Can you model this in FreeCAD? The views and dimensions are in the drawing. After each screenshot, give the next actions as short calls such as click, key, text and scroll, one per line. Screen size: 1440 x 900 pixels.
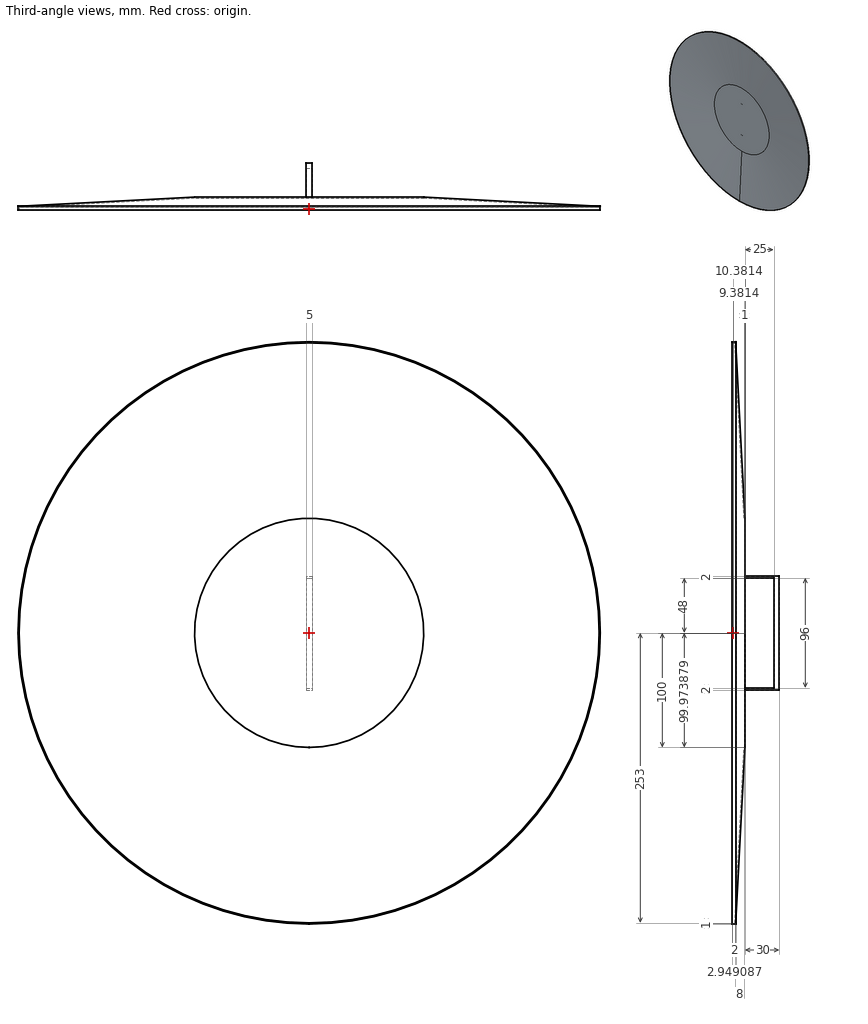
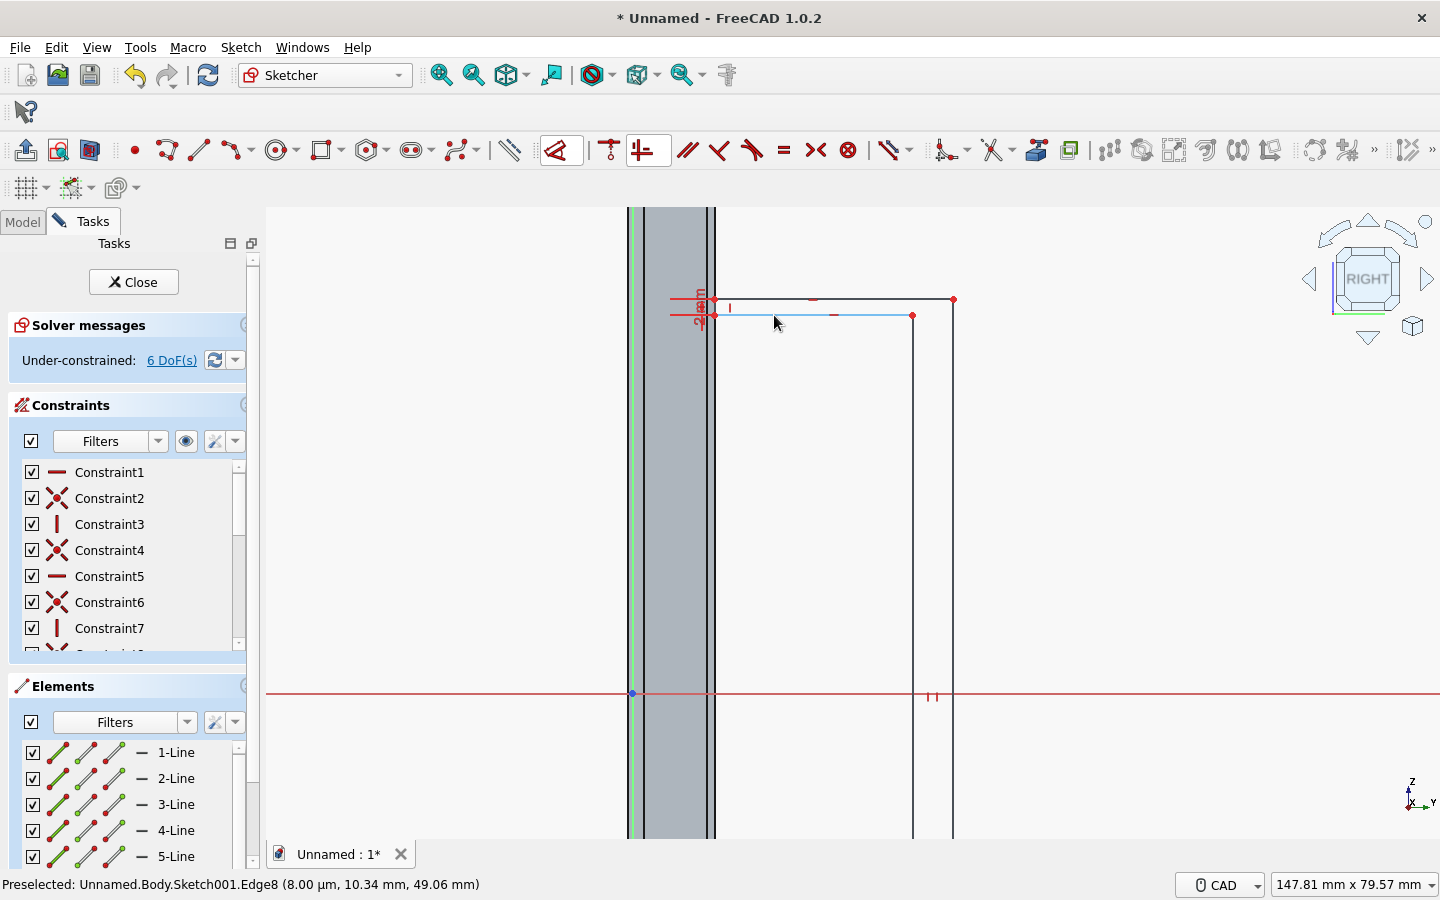
click(774, 315)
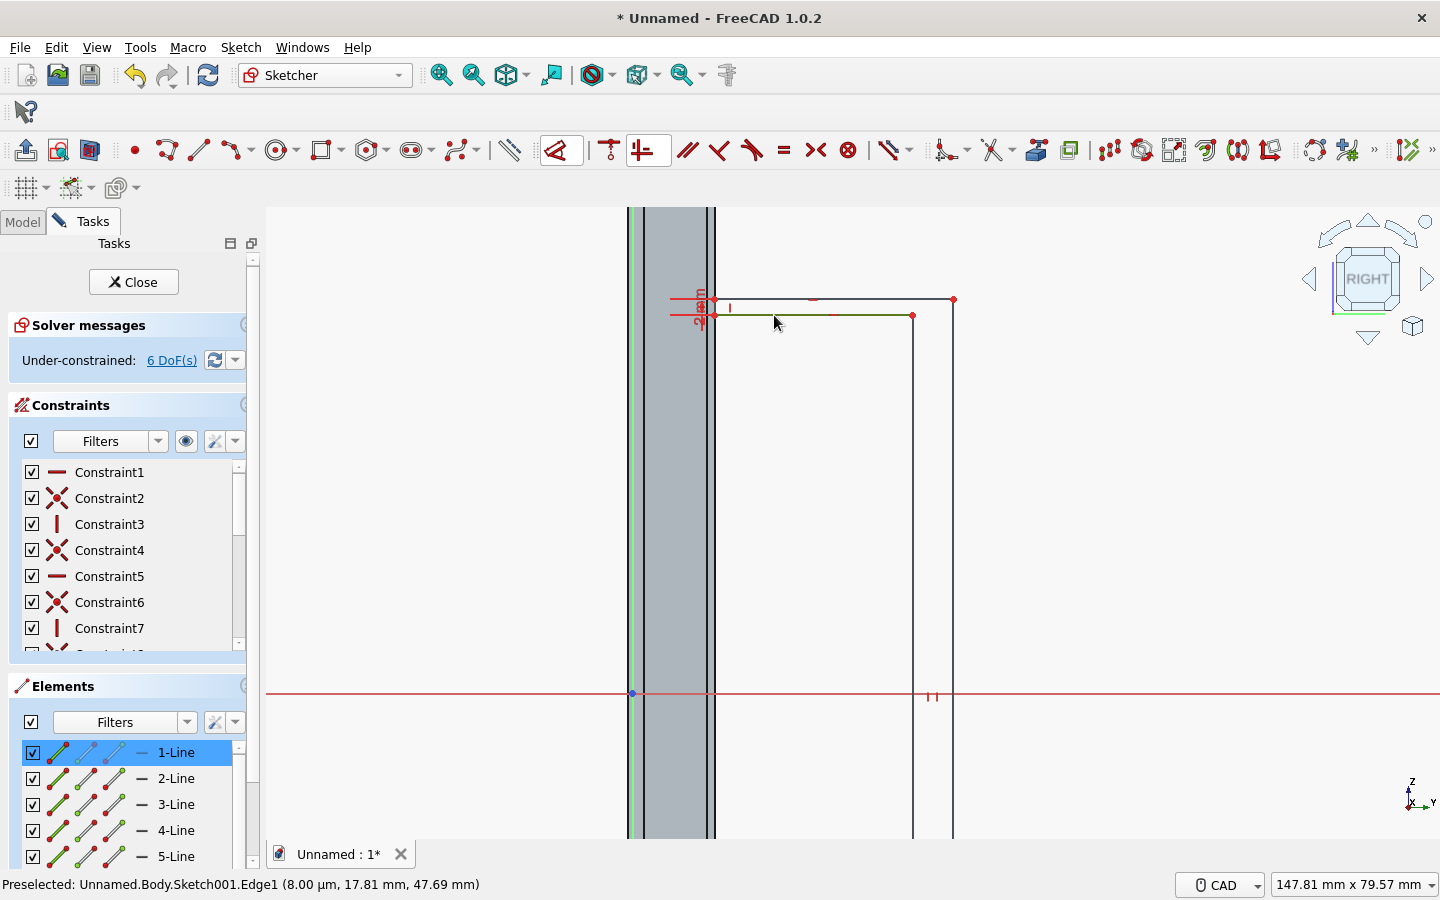
click(578, 150)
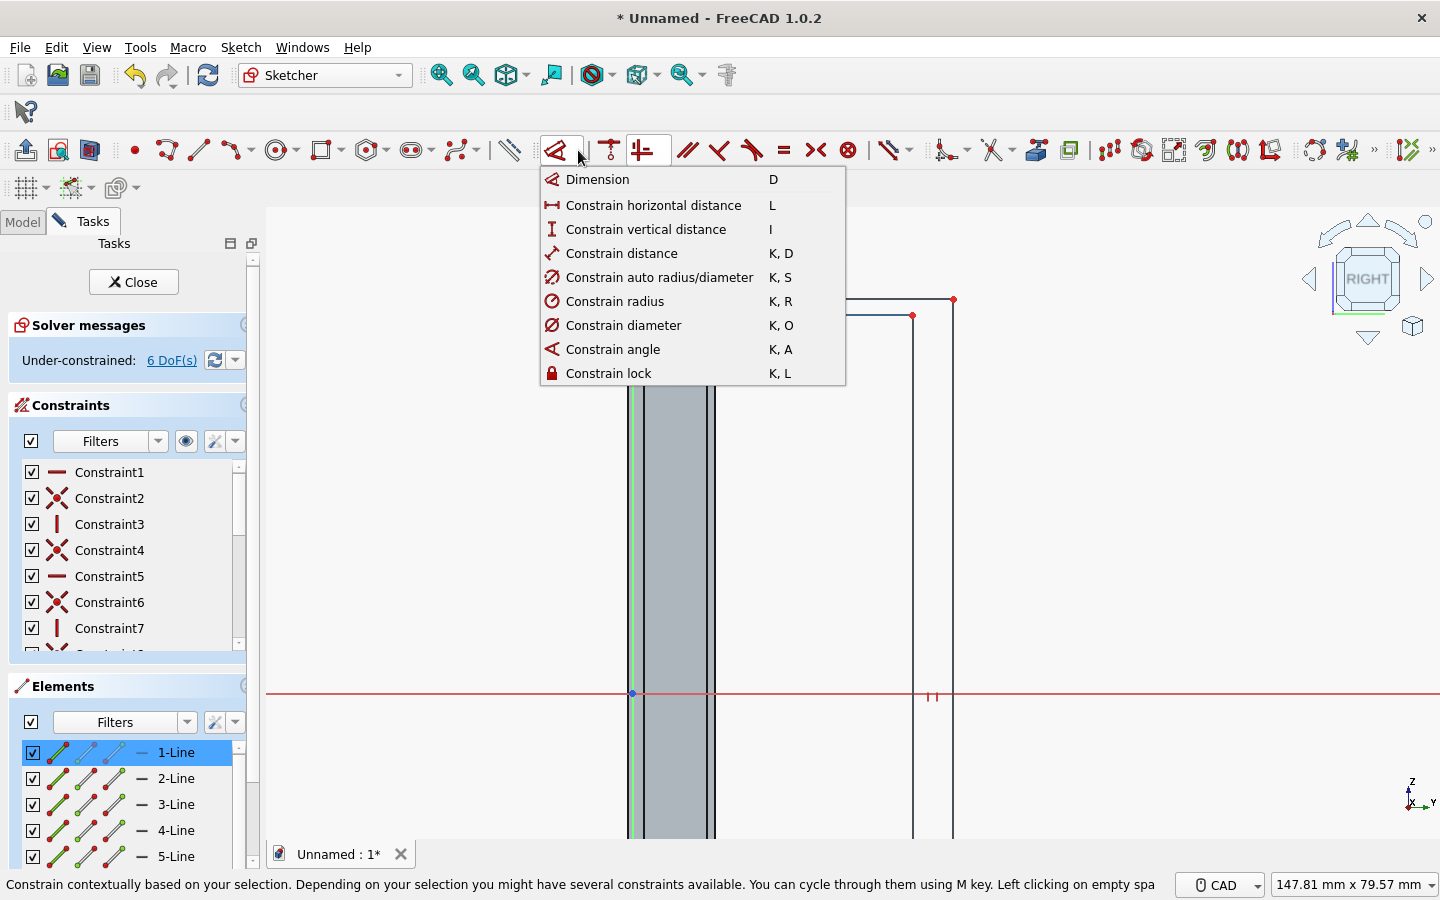
click(693, 205)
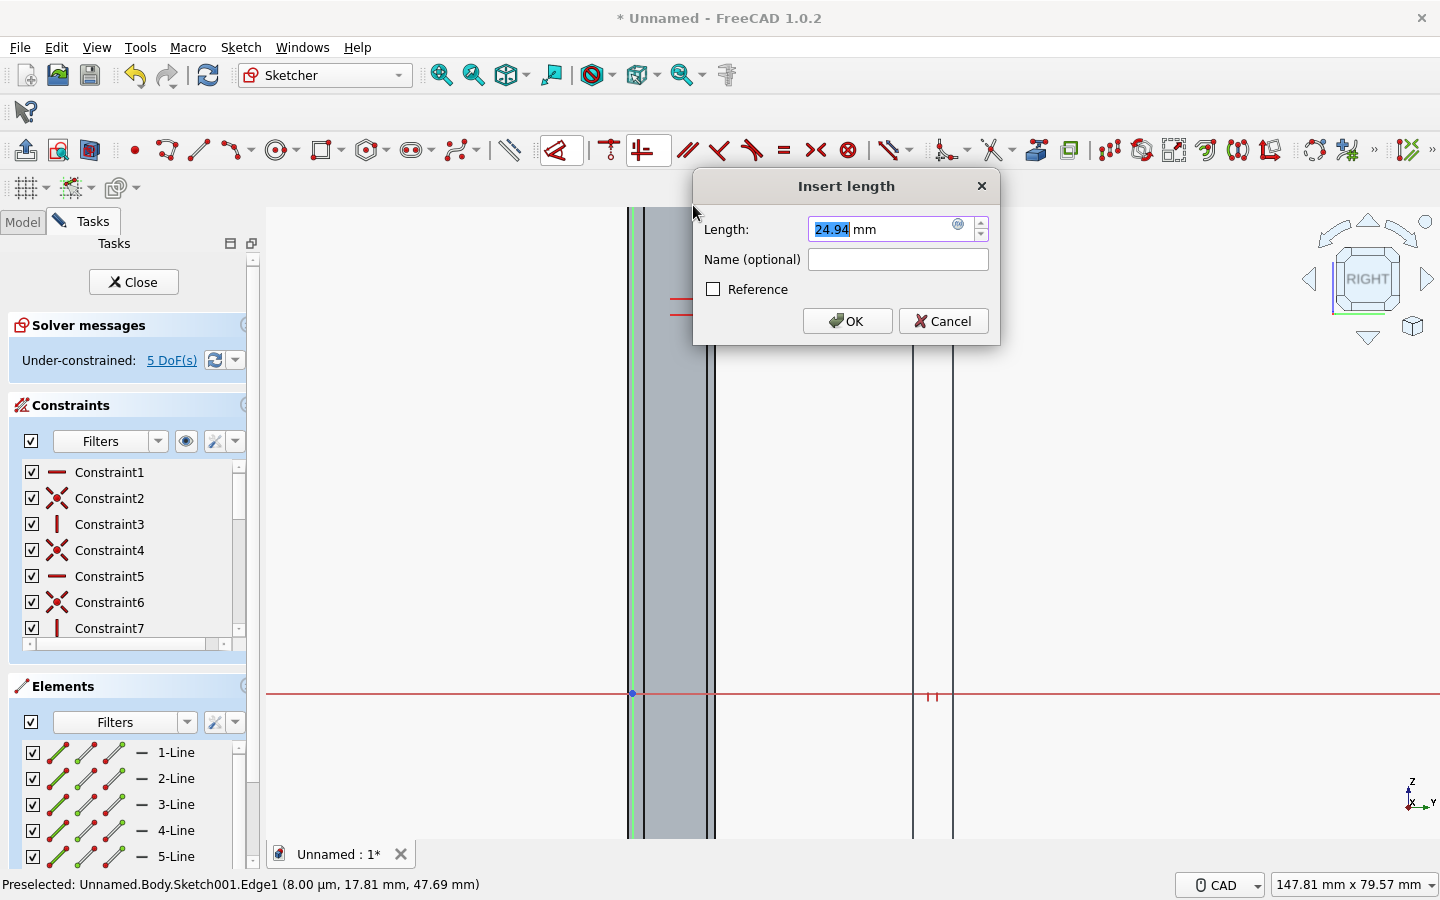
text(25)
key(Return)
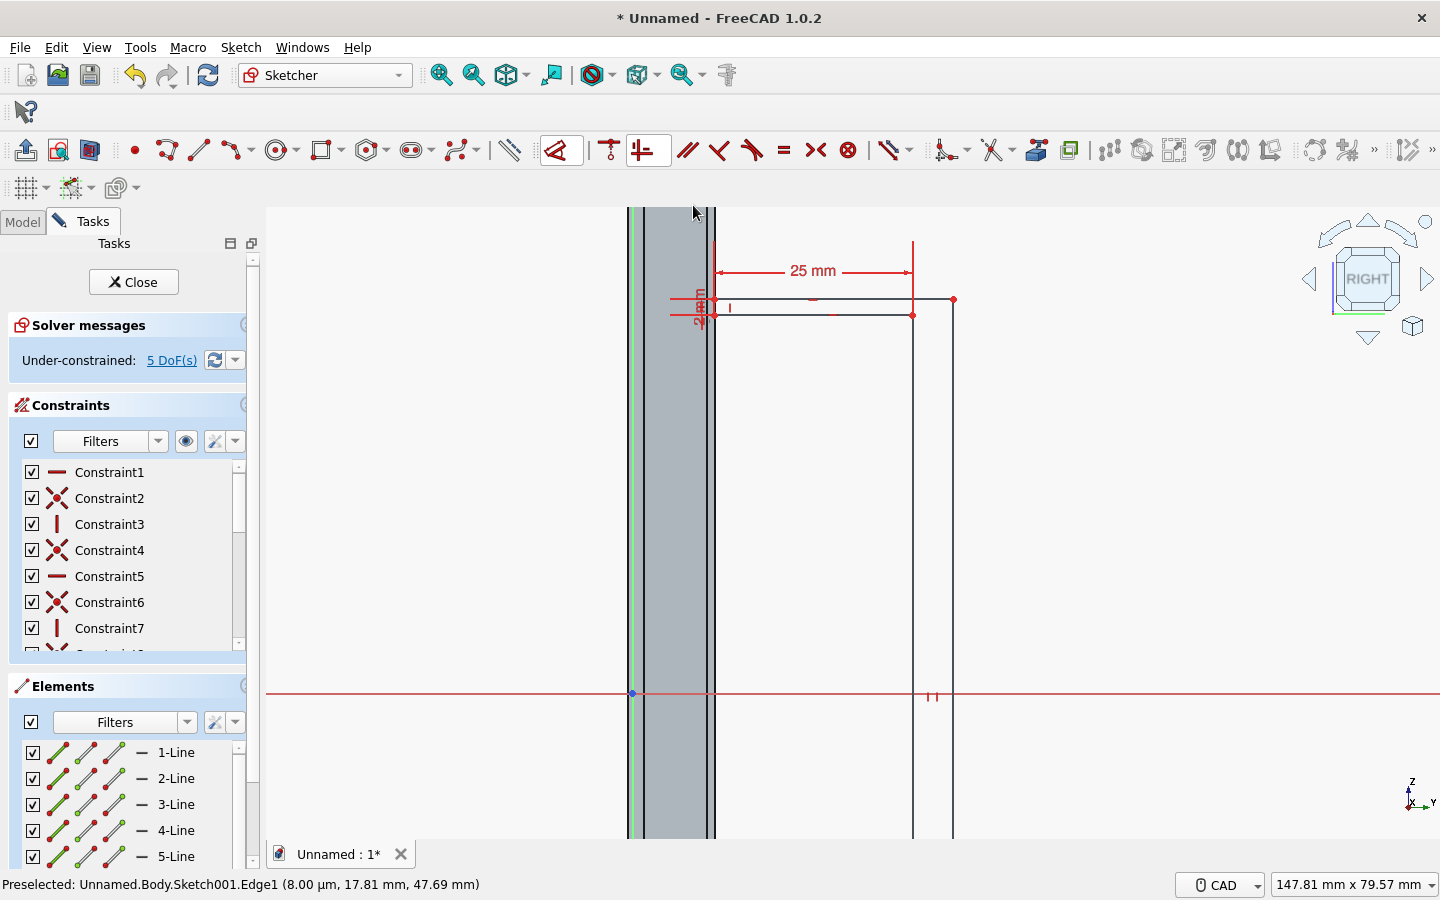
click(913, 544)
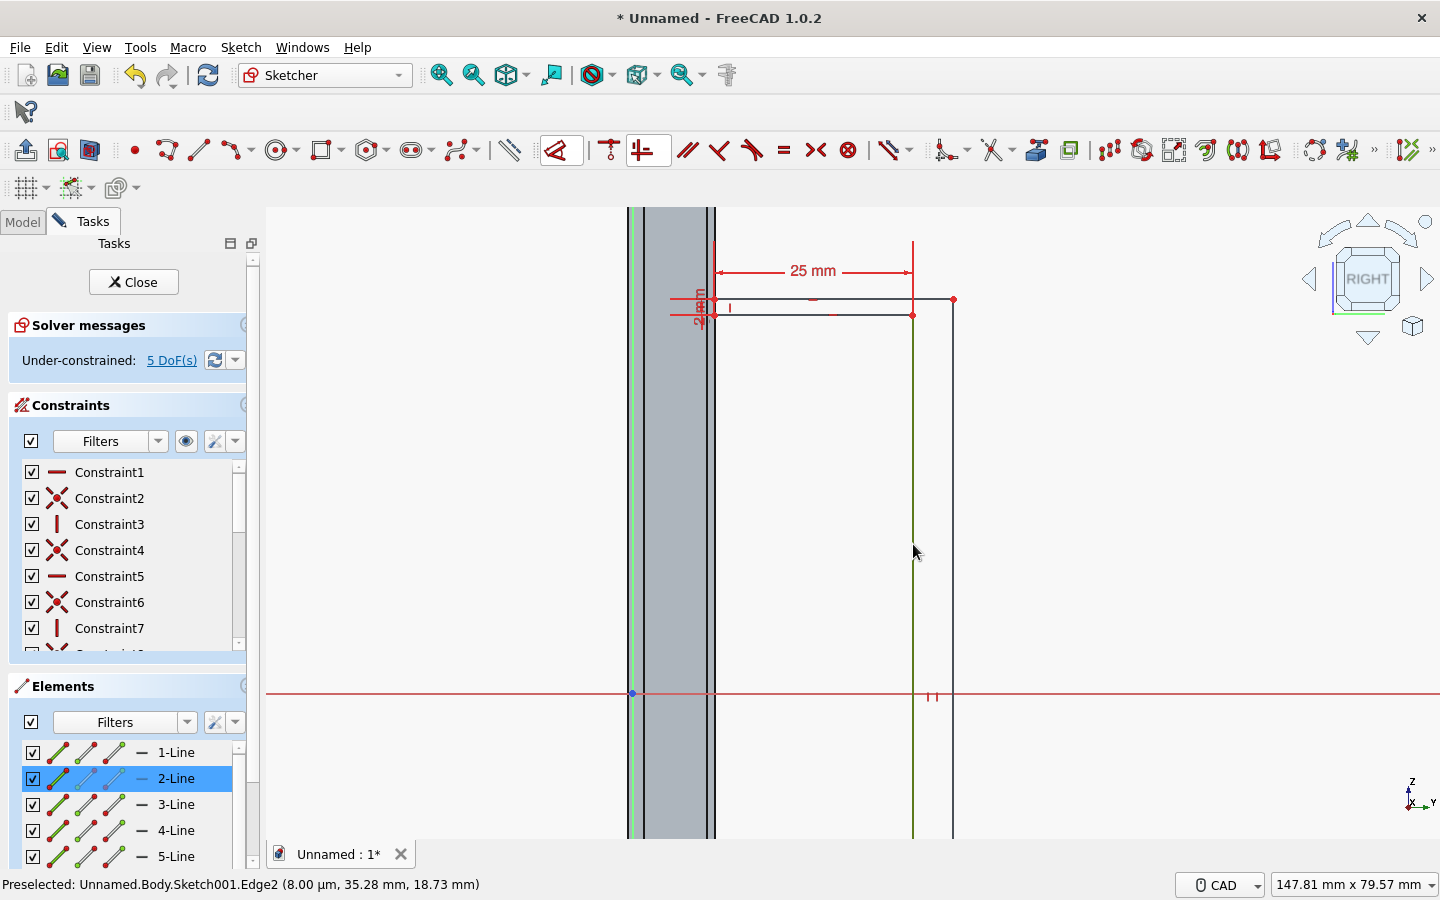
key(i)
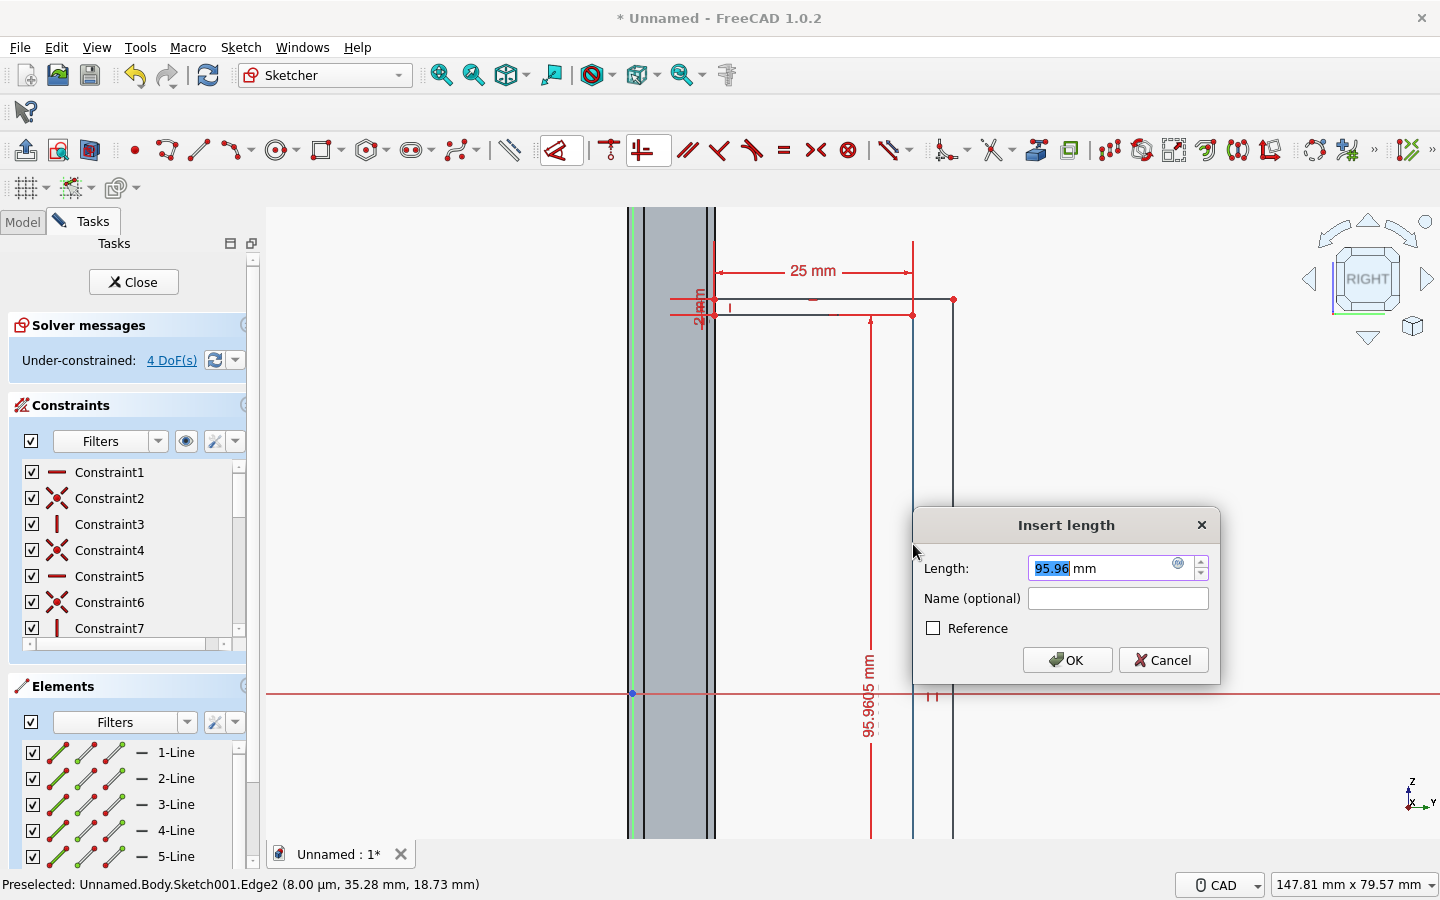
text(96)
key(Return)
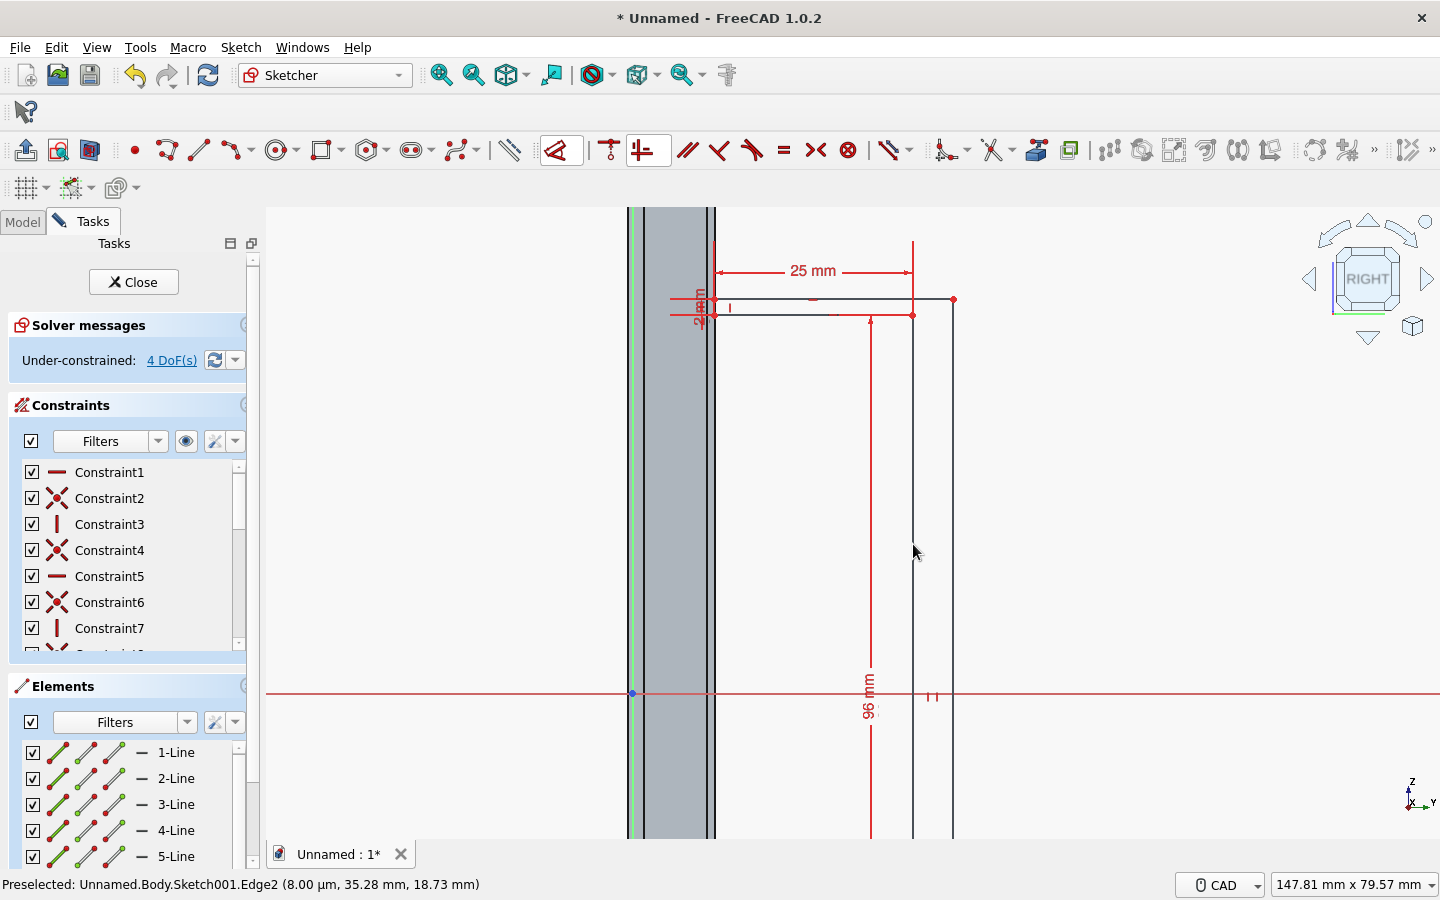
scroll(774, 315, down, 3)